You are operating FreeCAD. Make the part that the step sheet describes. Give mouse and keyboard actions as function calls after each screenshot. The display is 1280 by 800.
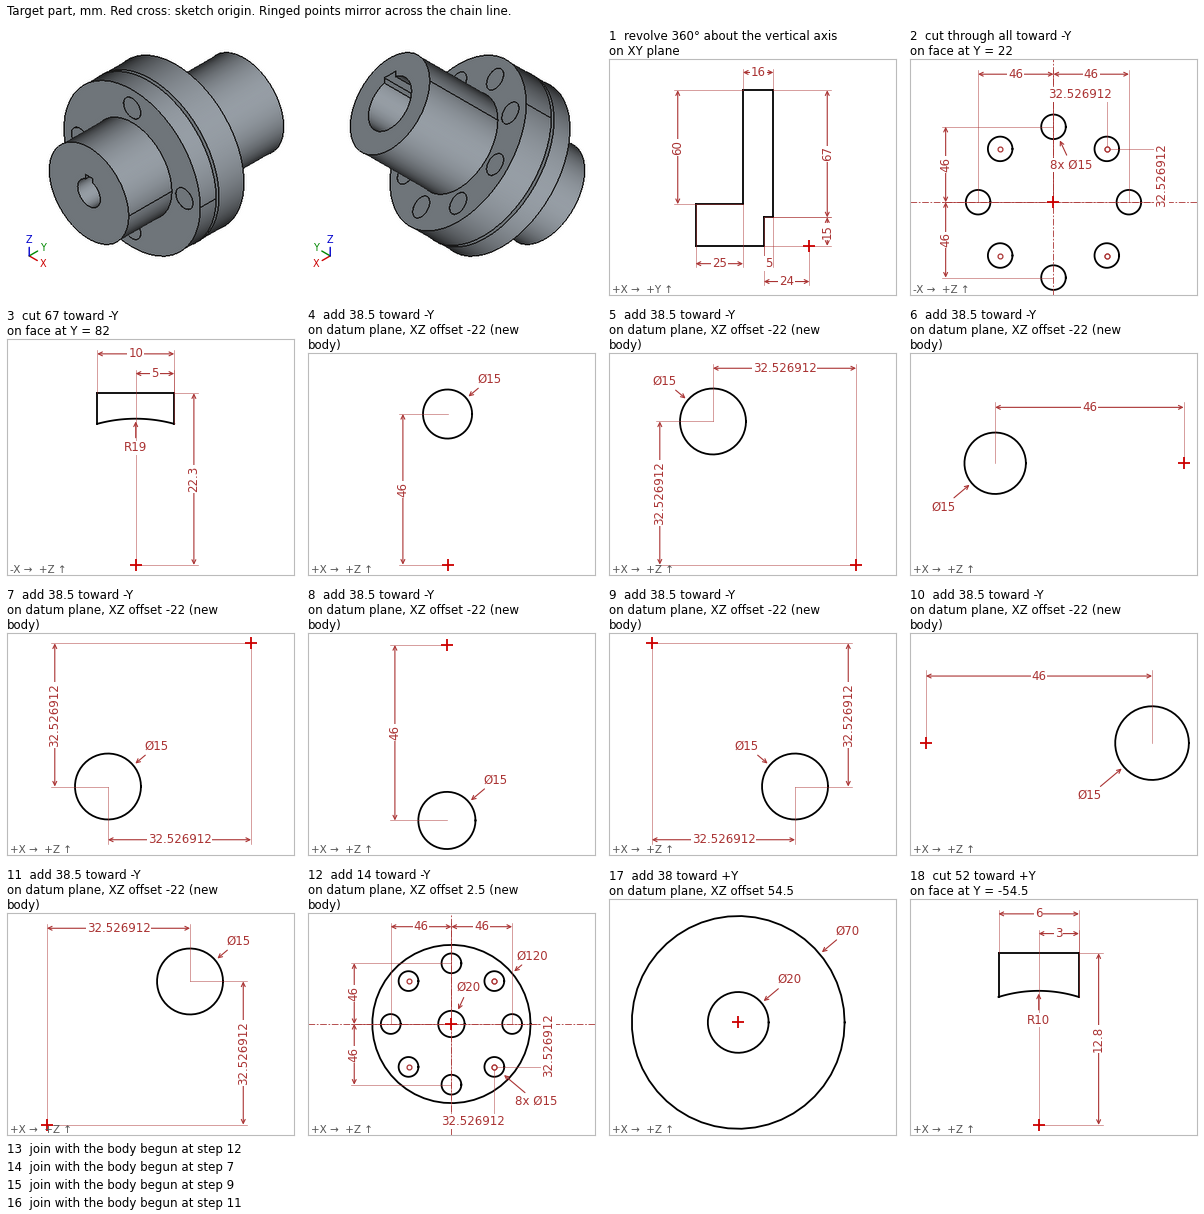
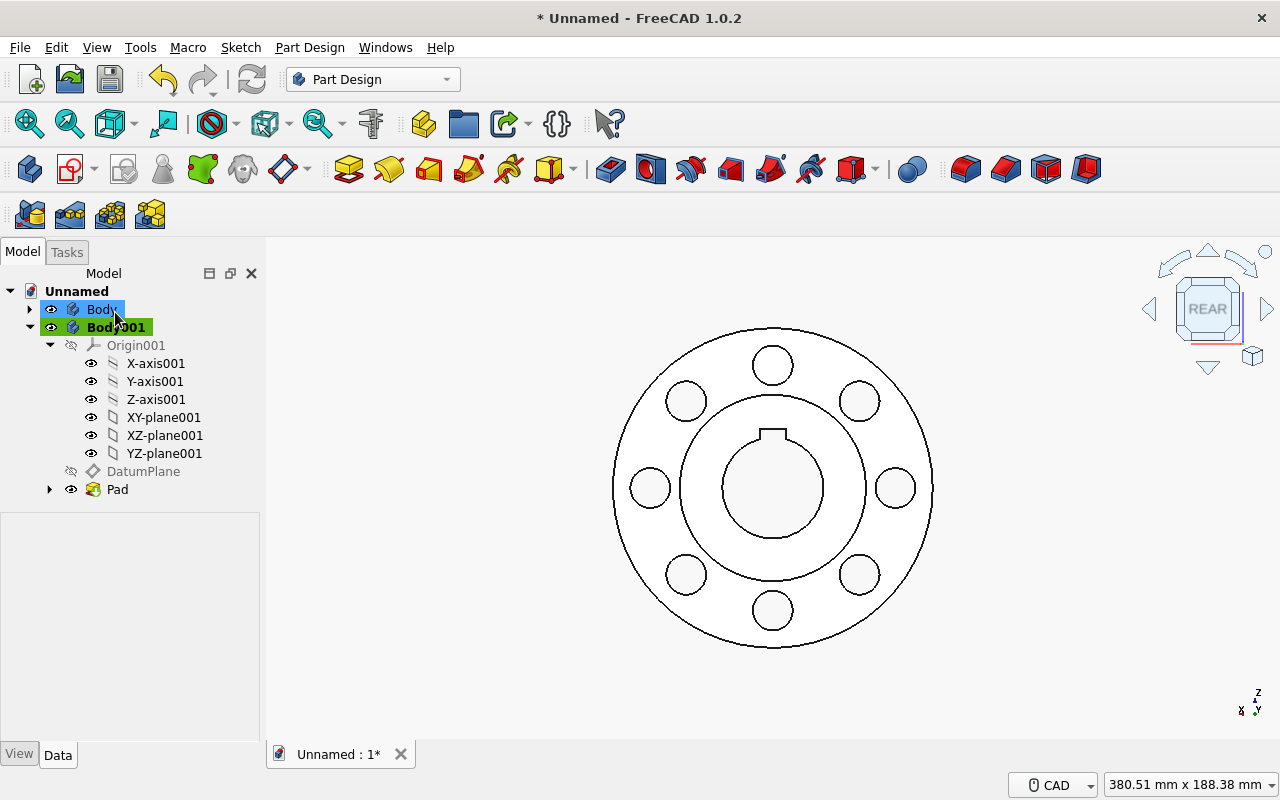
click(30, 124)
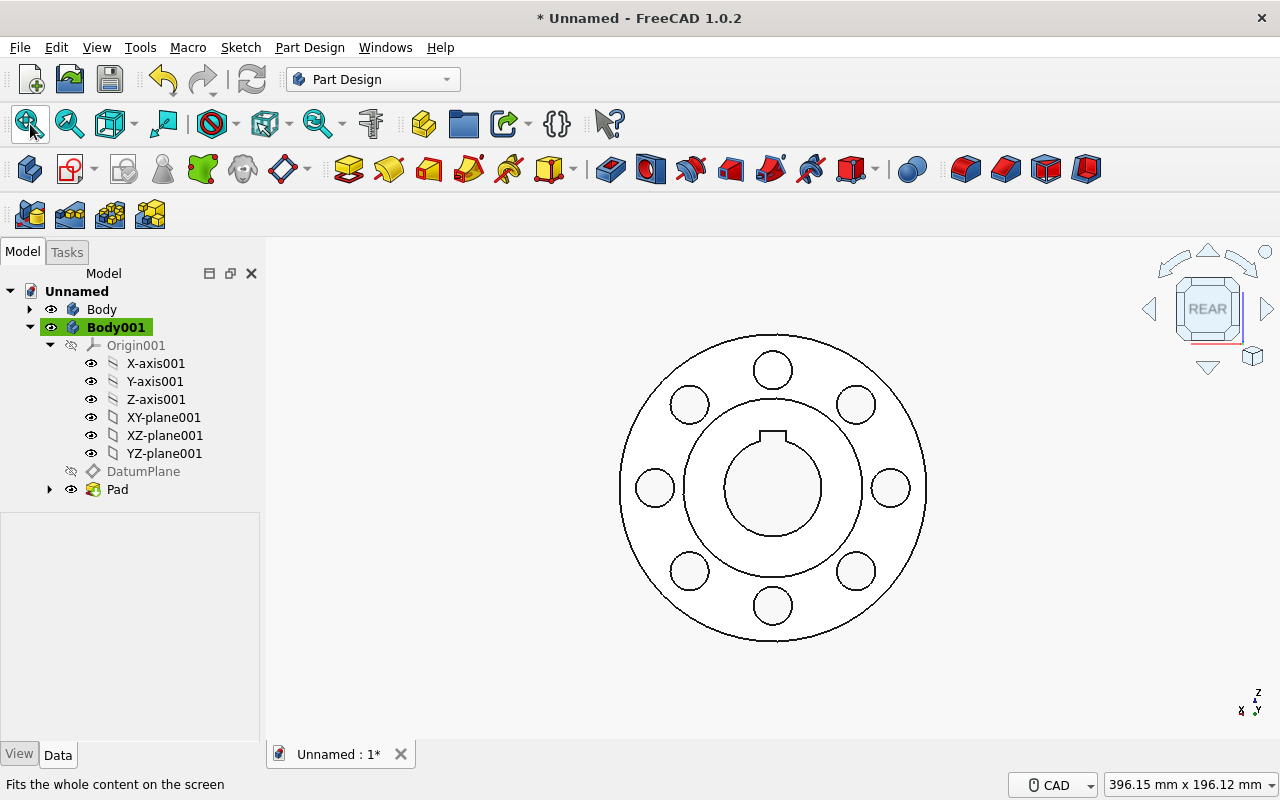
click(30, 170)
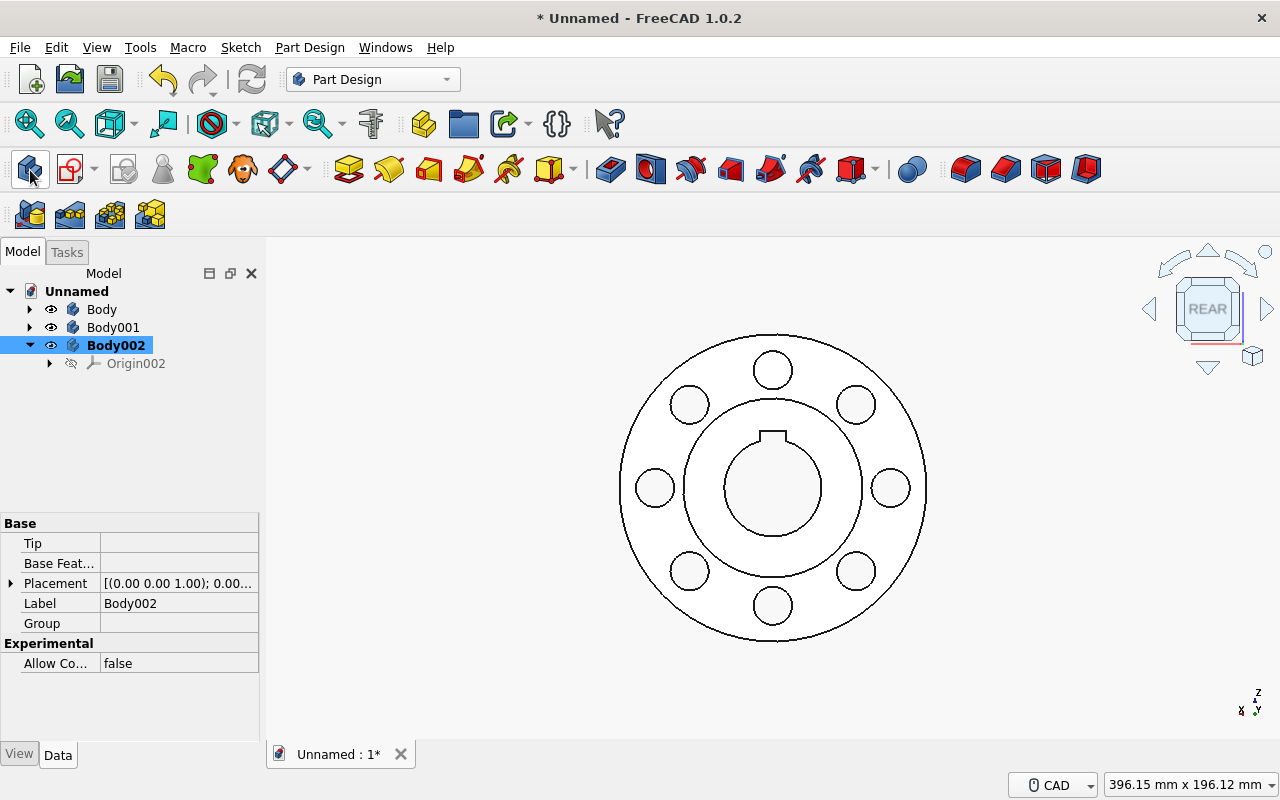
click(50, 363)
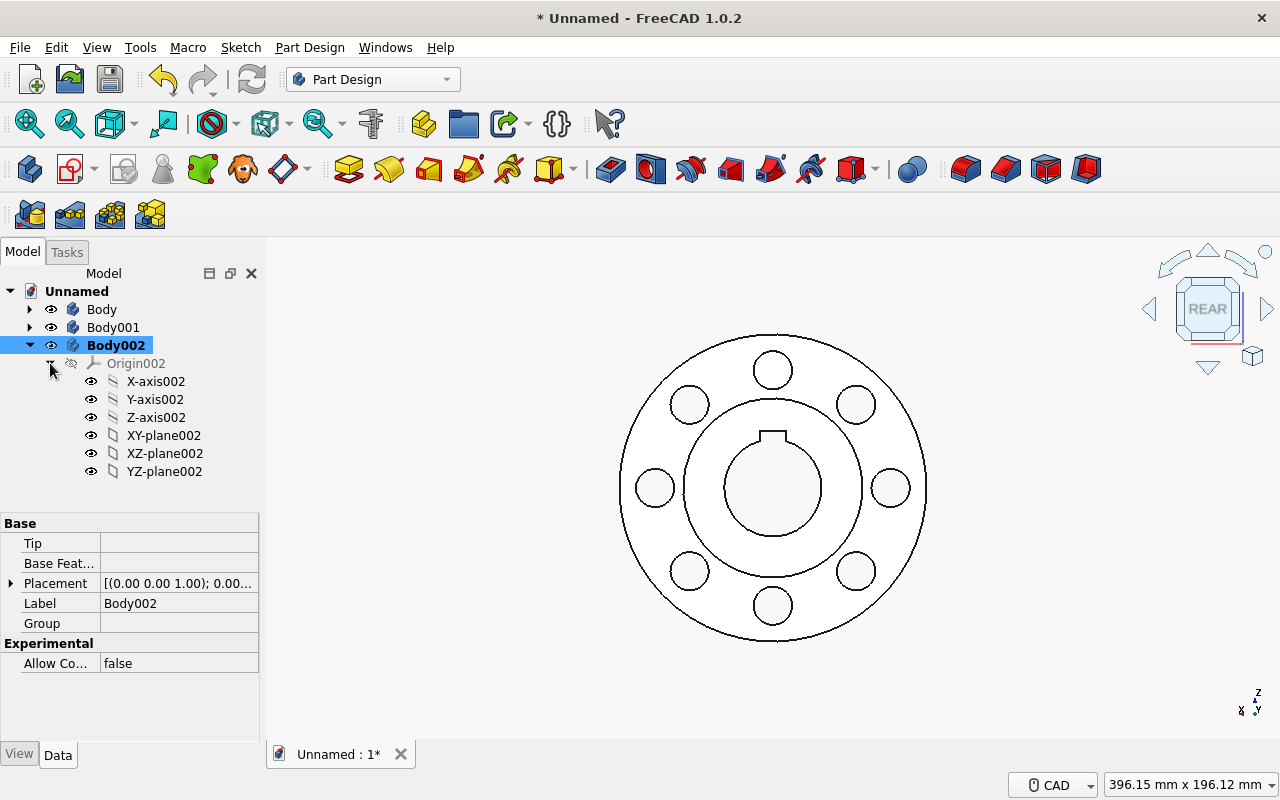
click(136, 453)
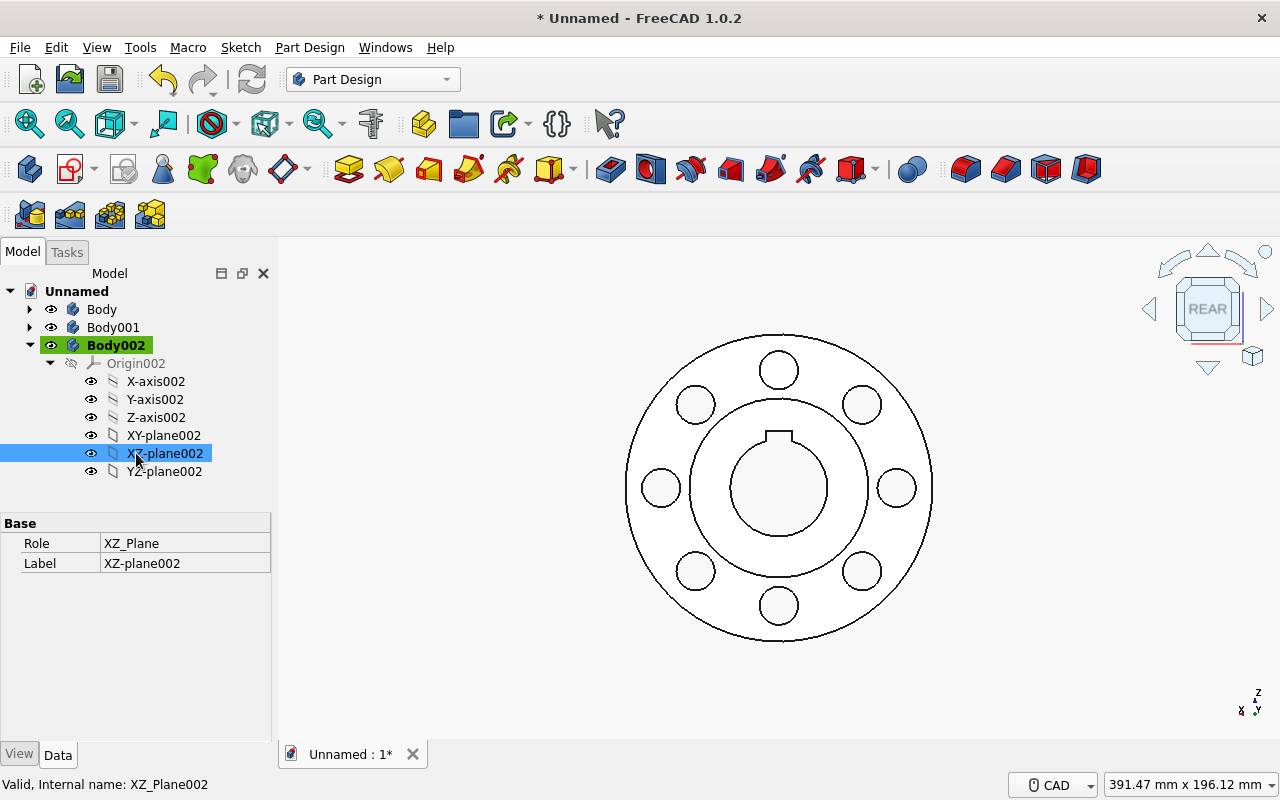
click(284, 170)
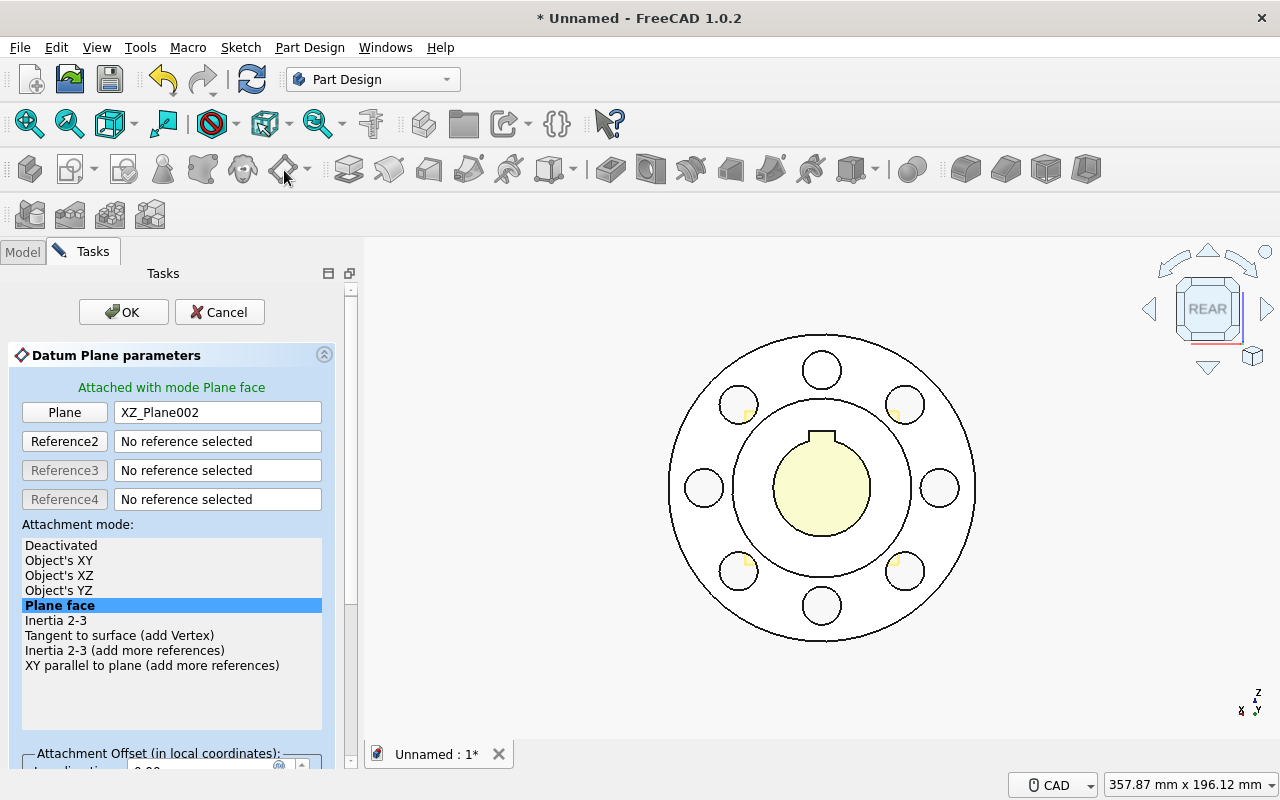
scroll(351, 526, down, 3)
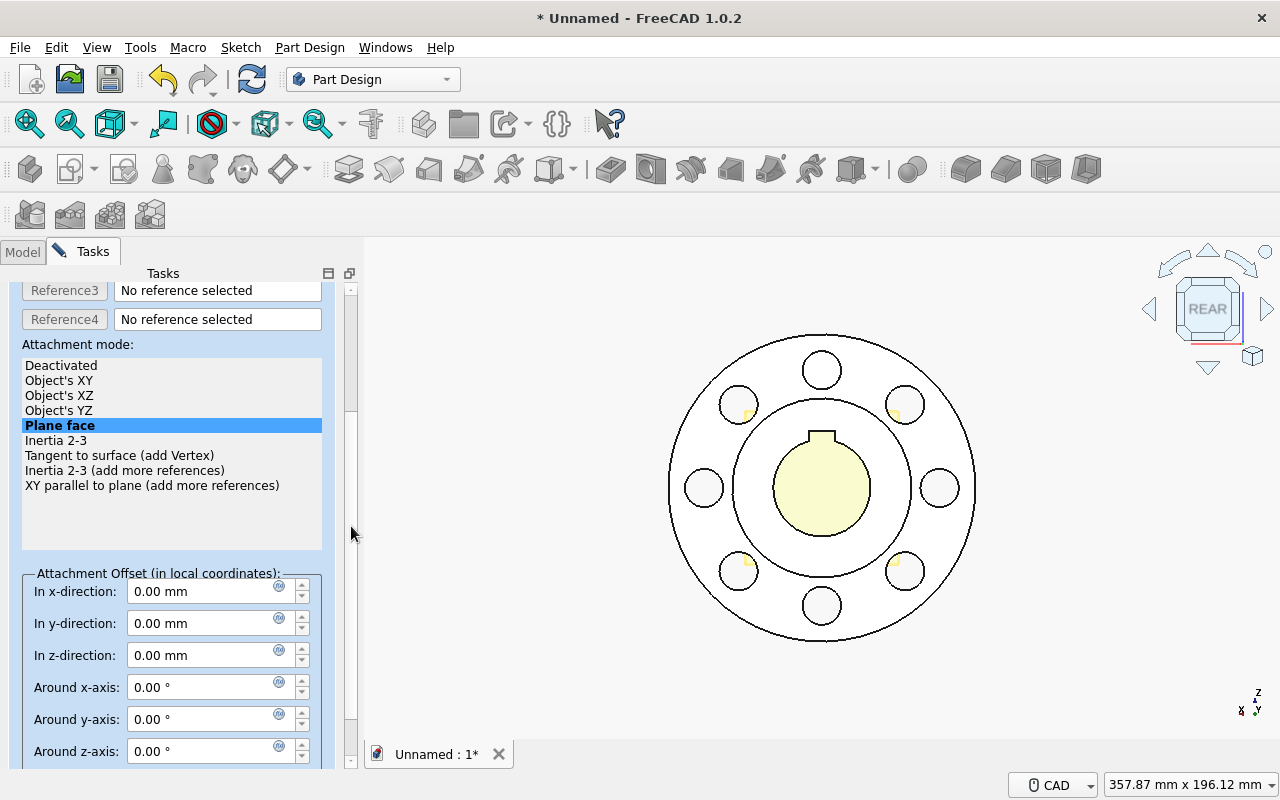
triple_click(210, 655)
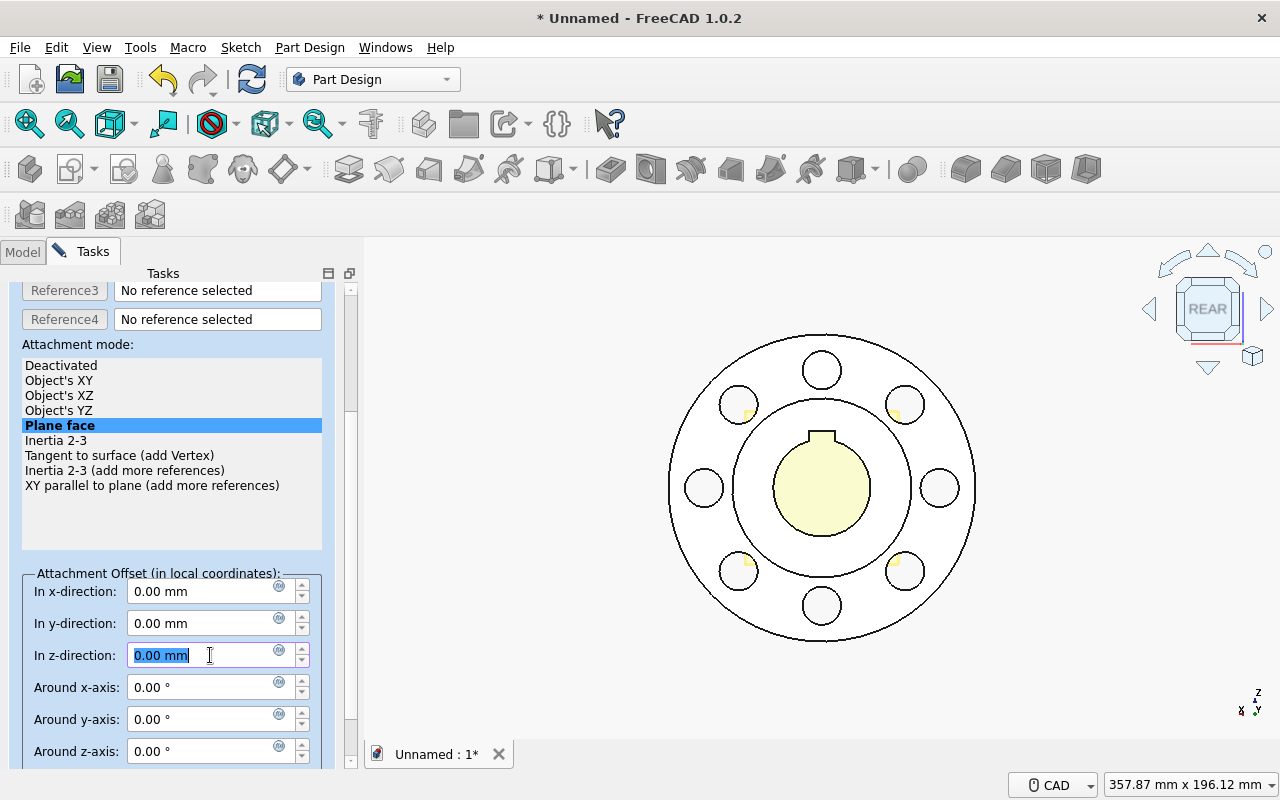
text(-22)
key(Tab)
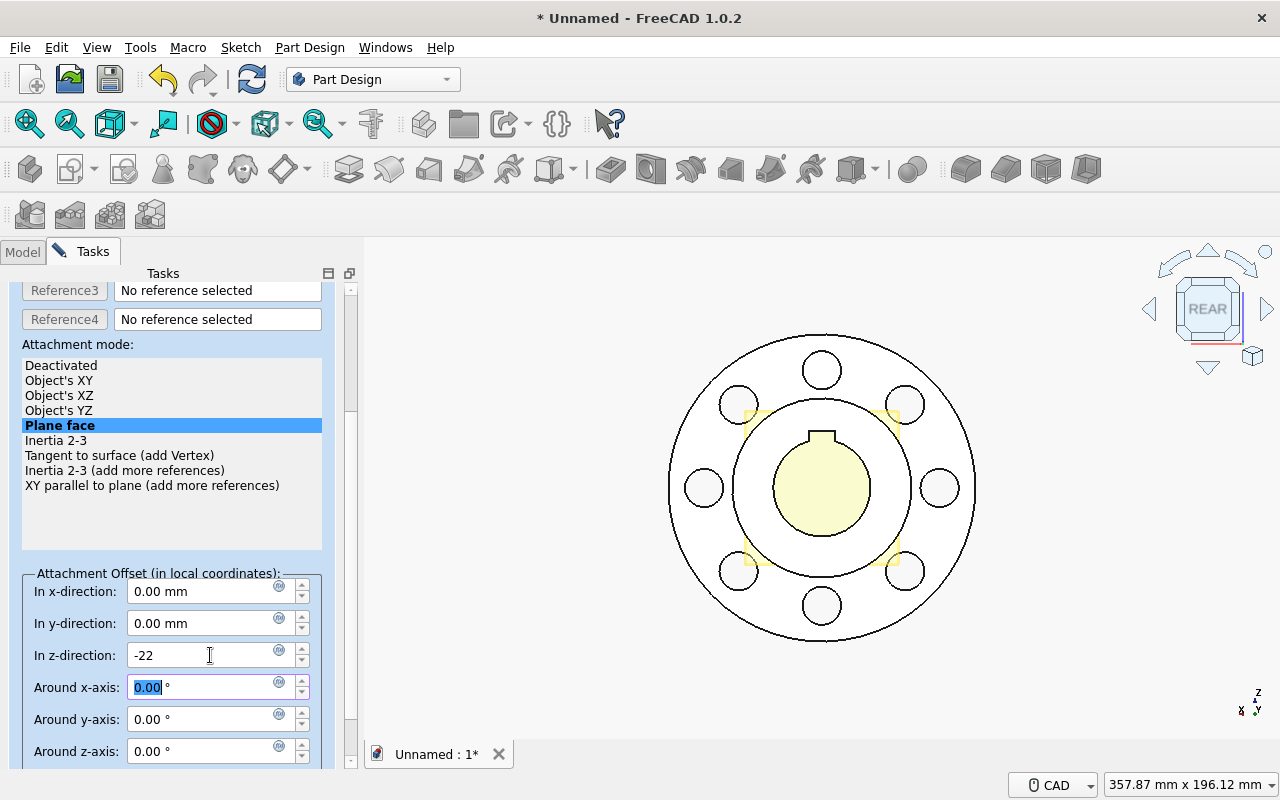
scroll(351, 526, up, 4)